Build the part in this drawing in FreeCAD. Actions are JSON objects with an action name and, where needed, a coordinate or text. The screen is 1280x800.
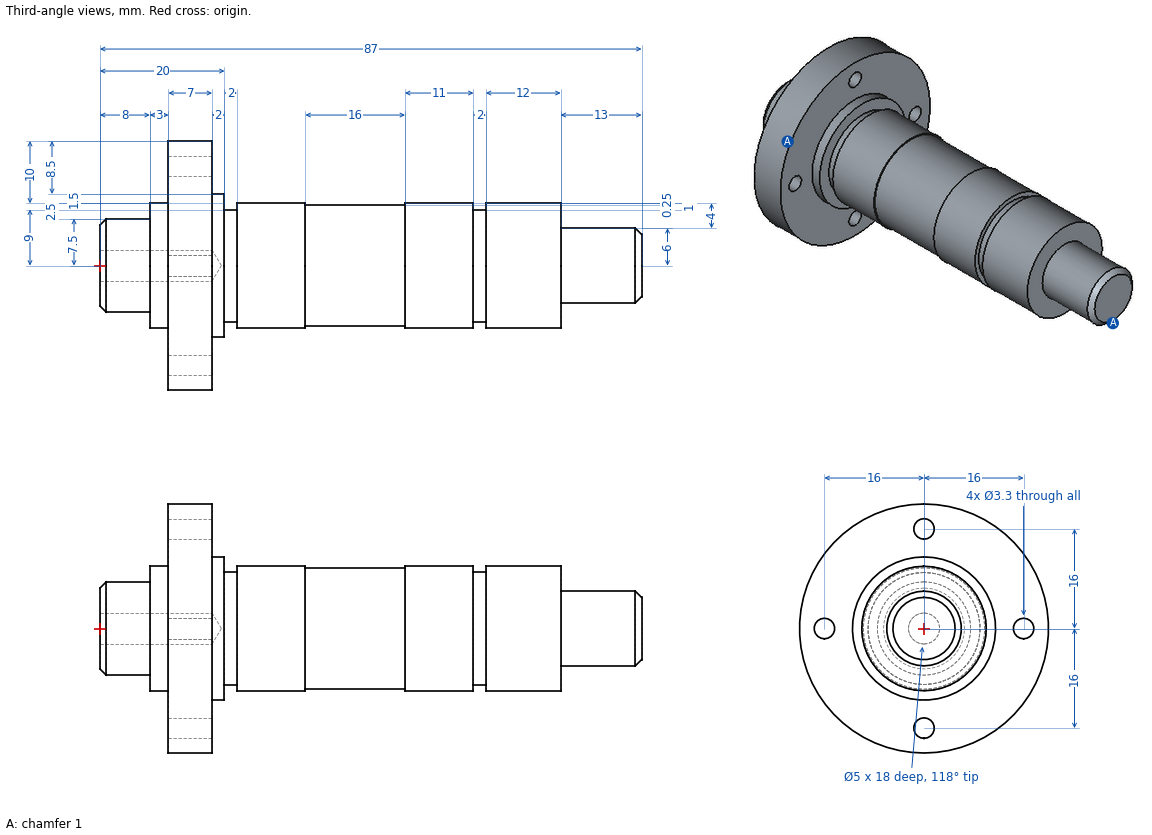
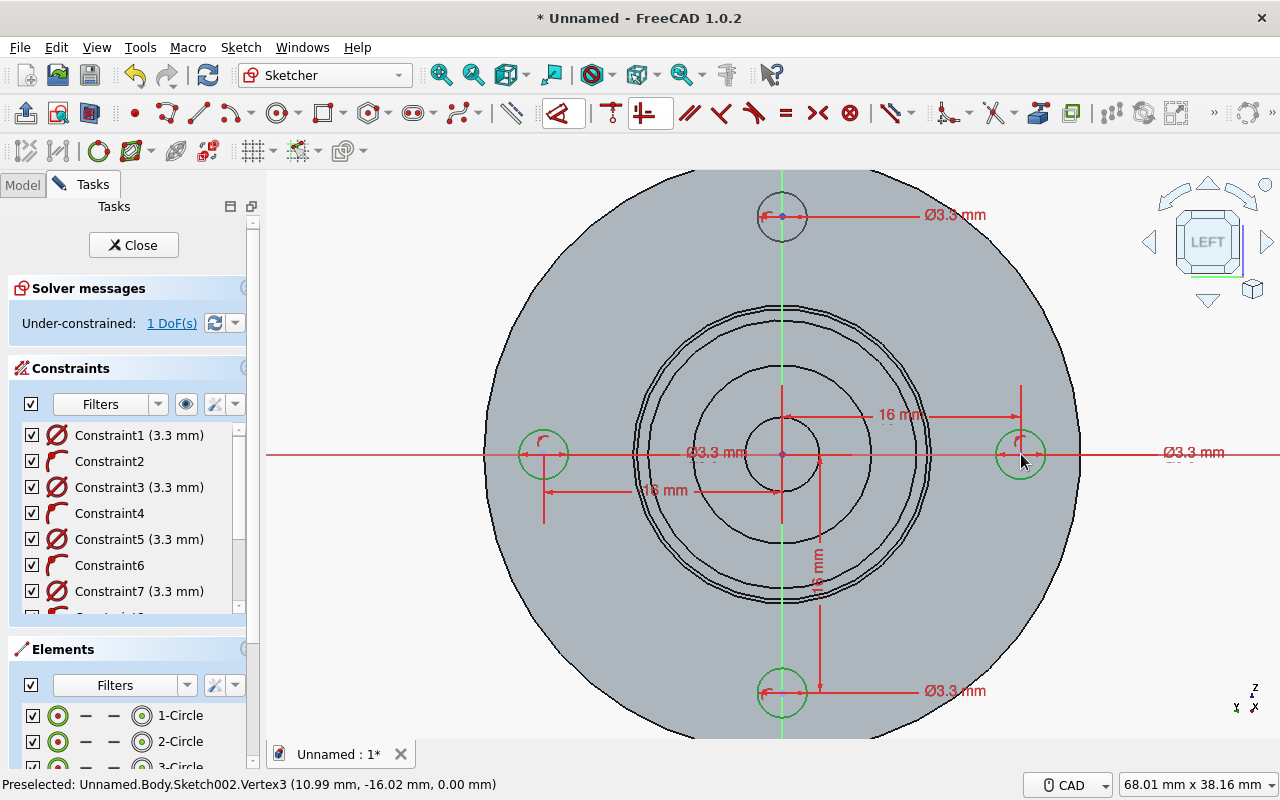
{"action": "left_click", "coordinate": [782, 217]}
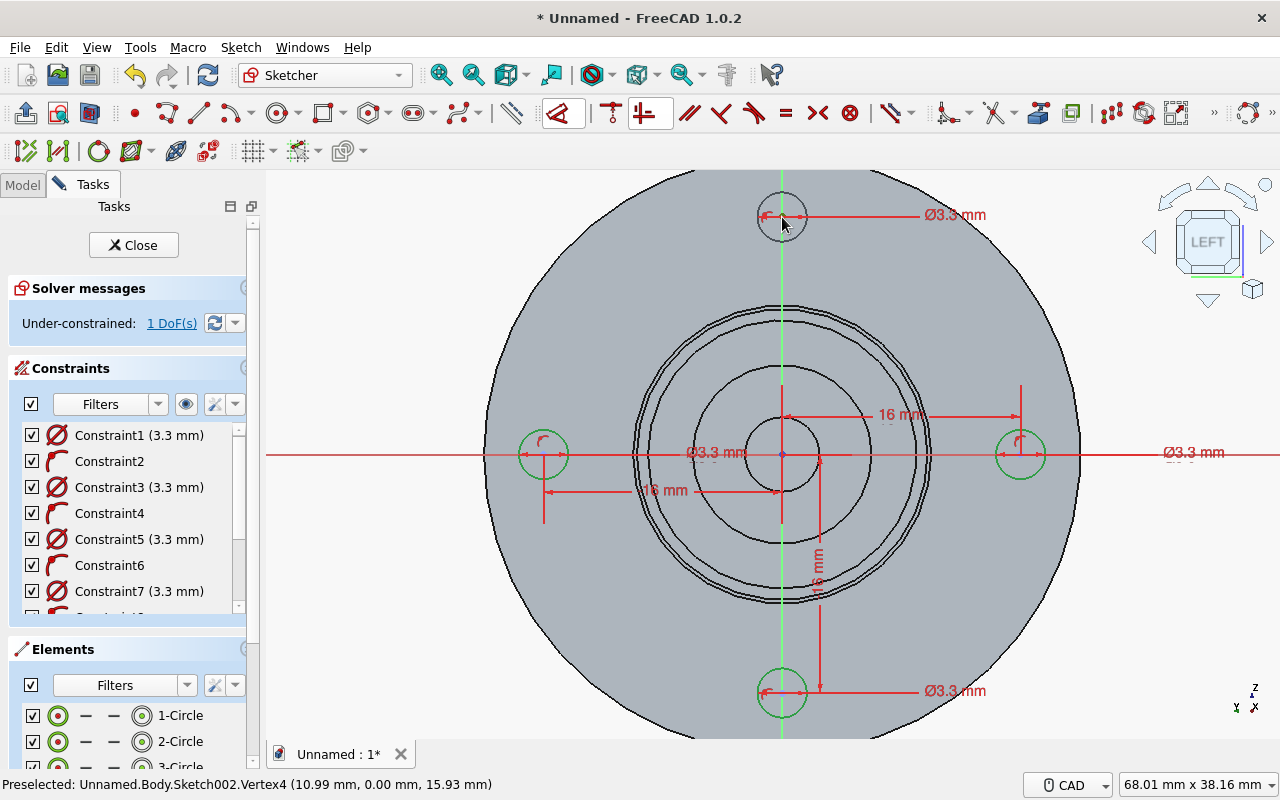
{"action": "key", "text": "i"}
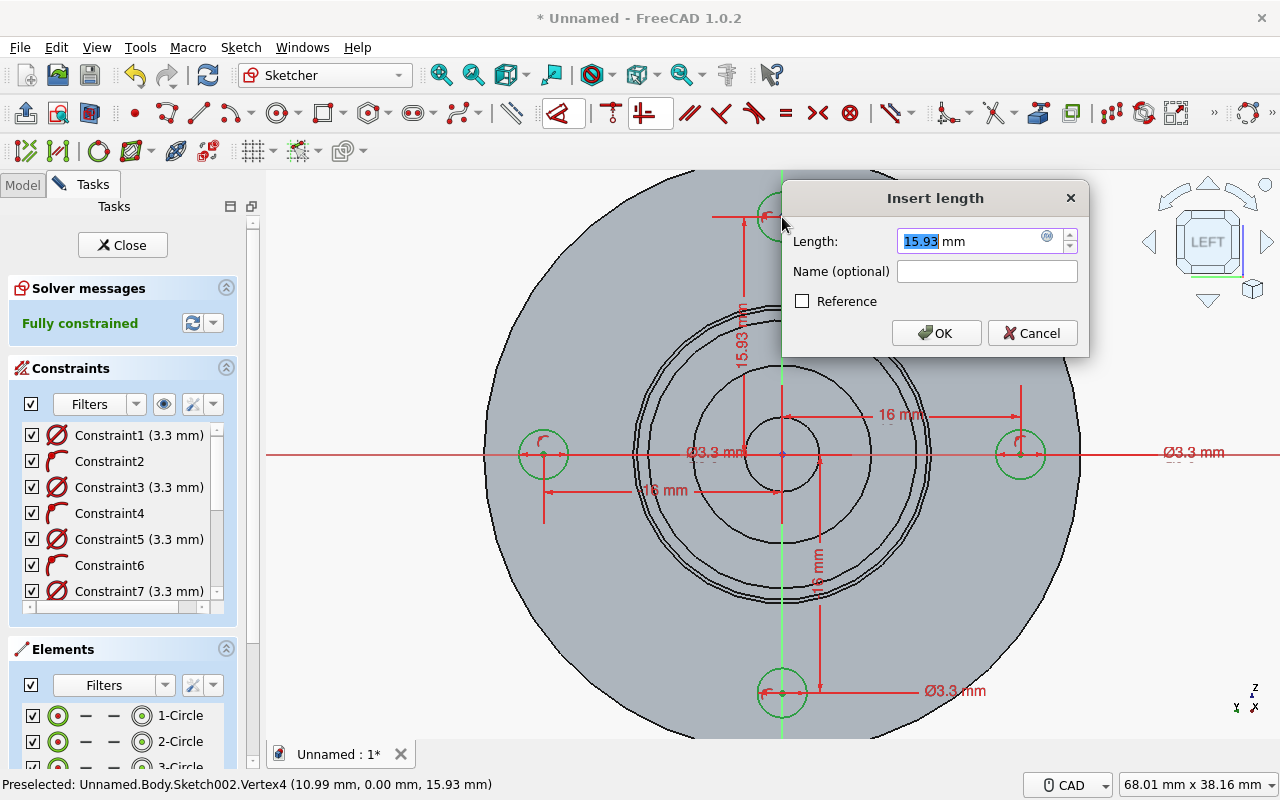
{"action": "type", "text": "16"}
{"action": "key", "text": "Return"}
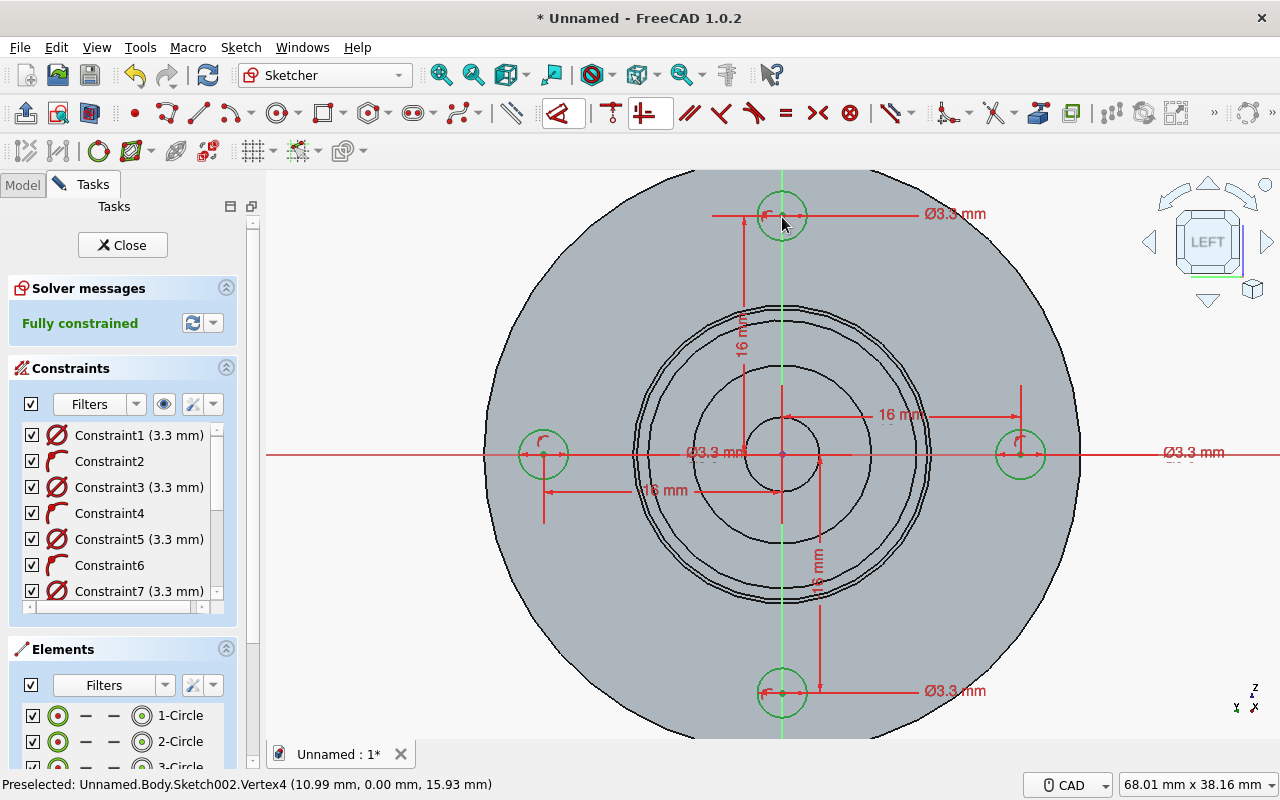
{"action": "left_click", "coordinate": [123, 245]}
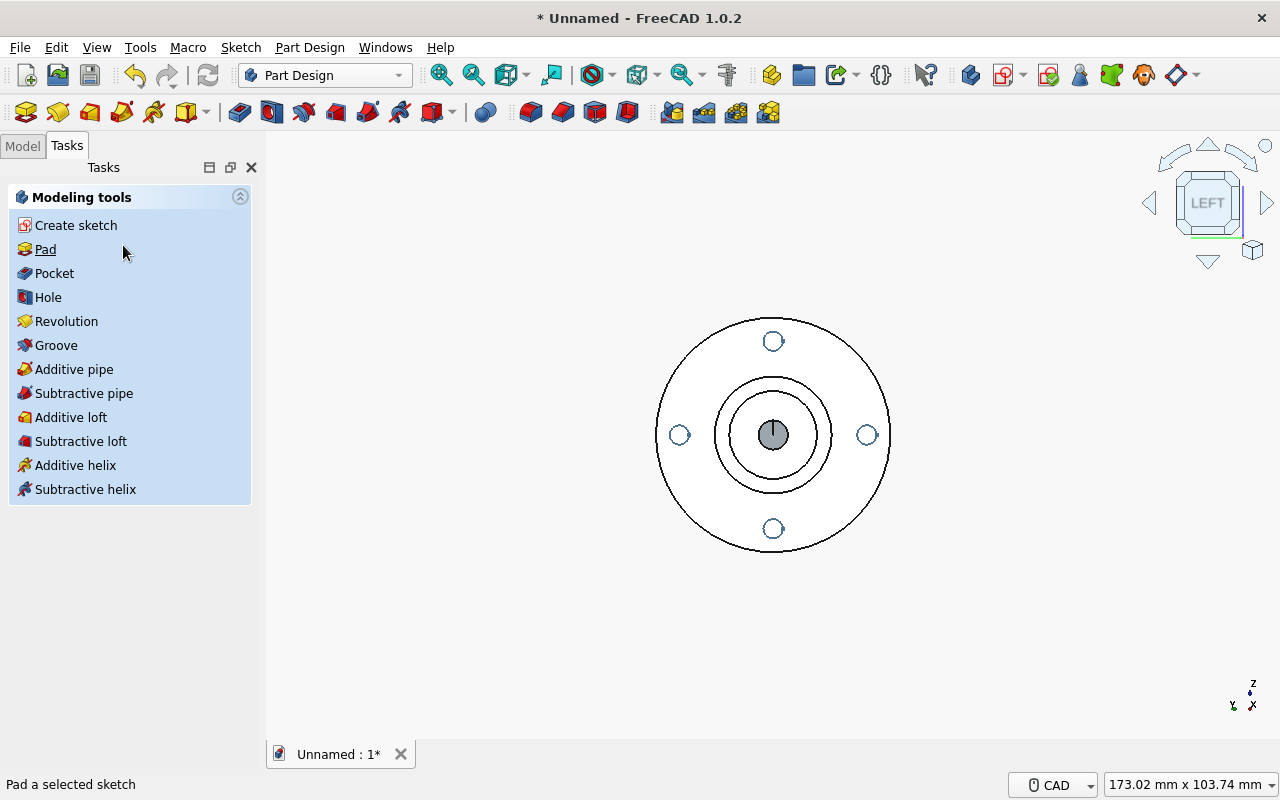
{"action": "left_click", "coordinate": [272, 112]}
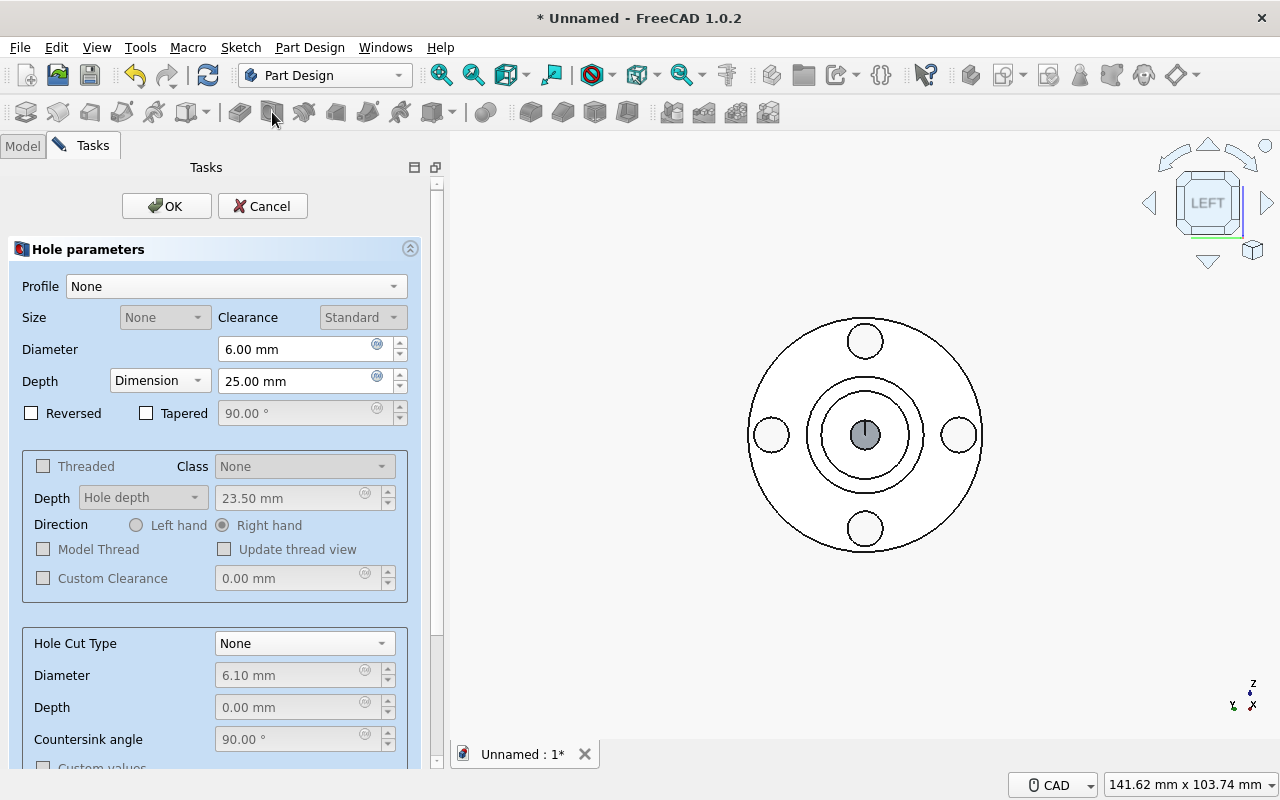
{"action": "triple_click", "coordinate": [305, 349]}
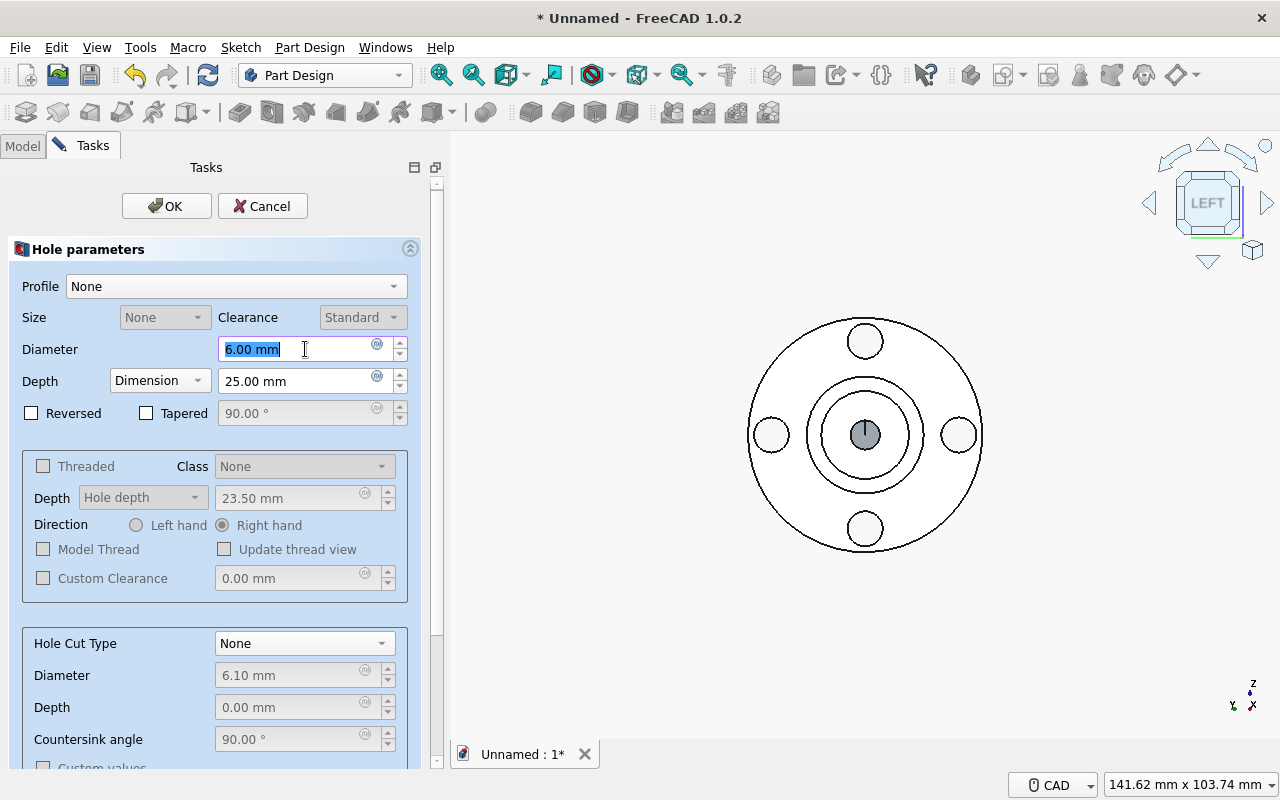
{"action": "type", "text": "3.3"}
{"action": "key", "text": "Tab"}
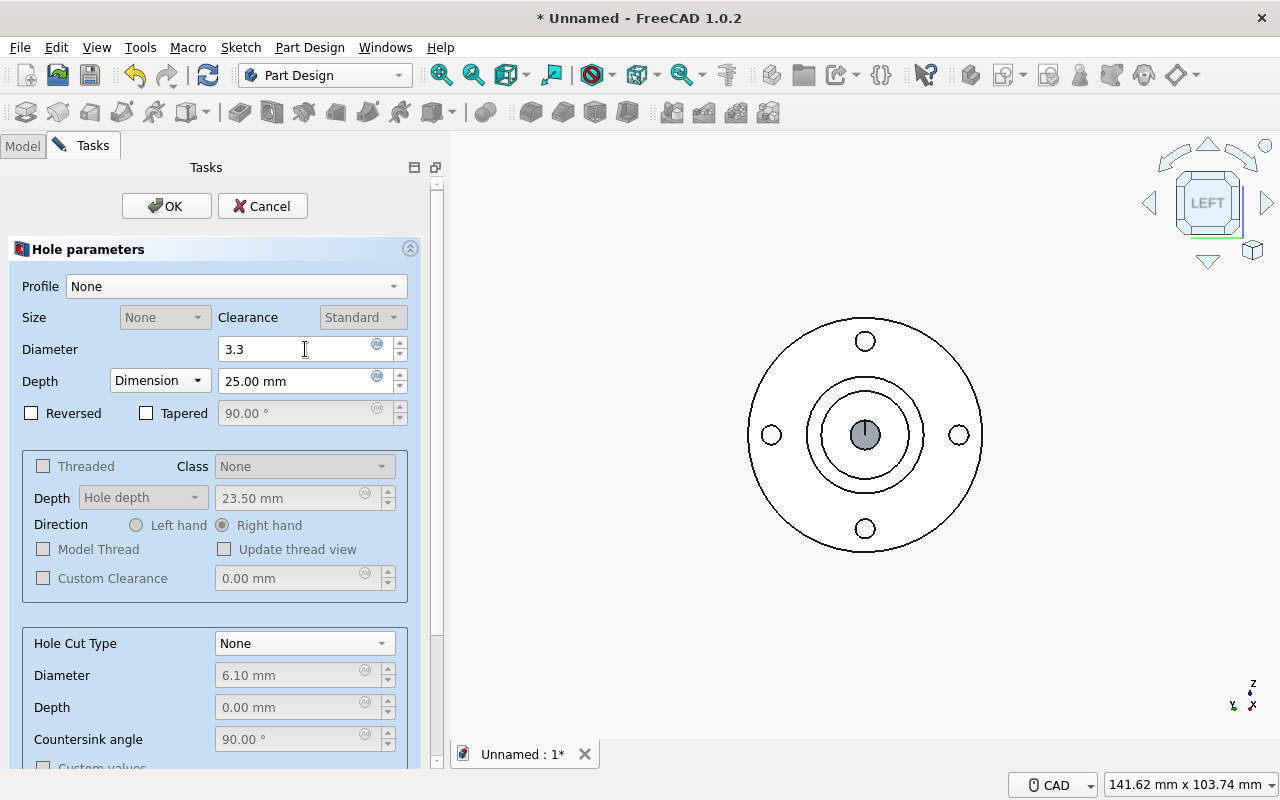
{"action": "left_click", "coordinate": [161, 380]}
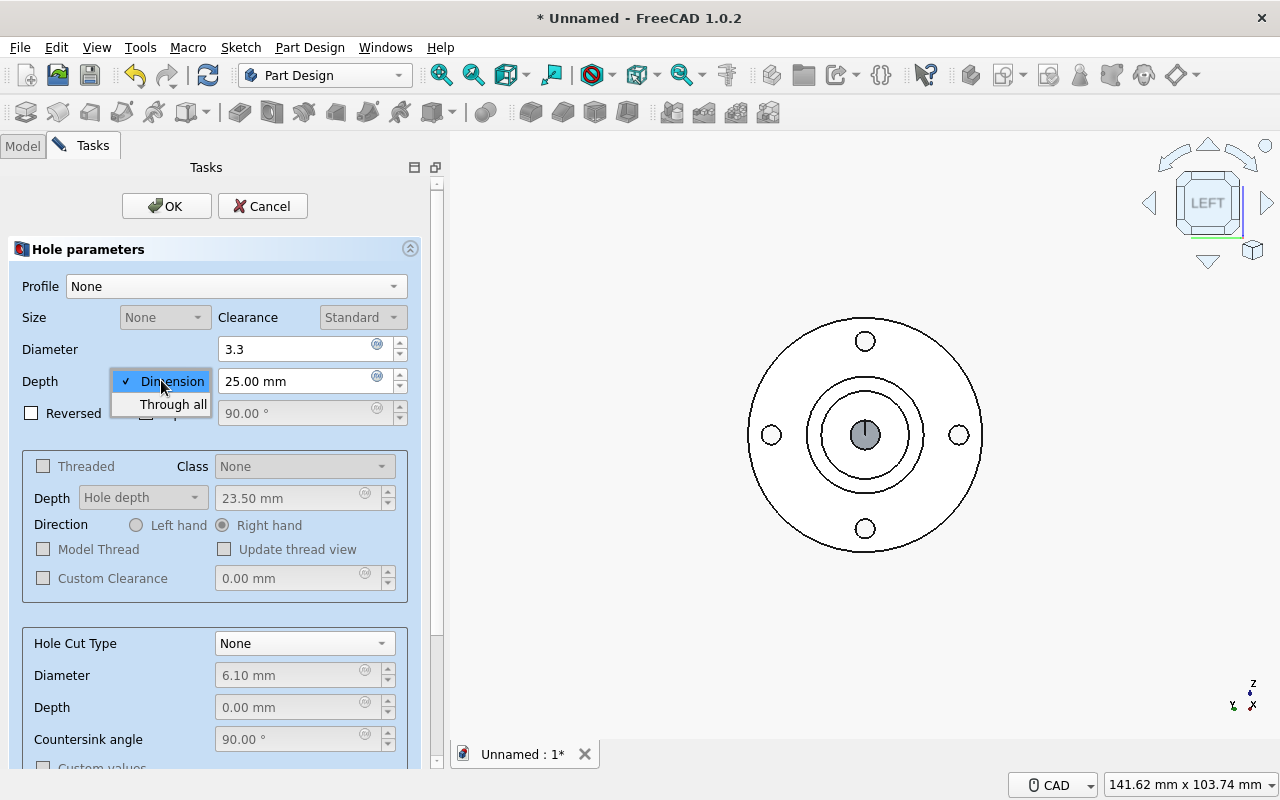
{"action": "left_click", "coordinate": [160, 404]}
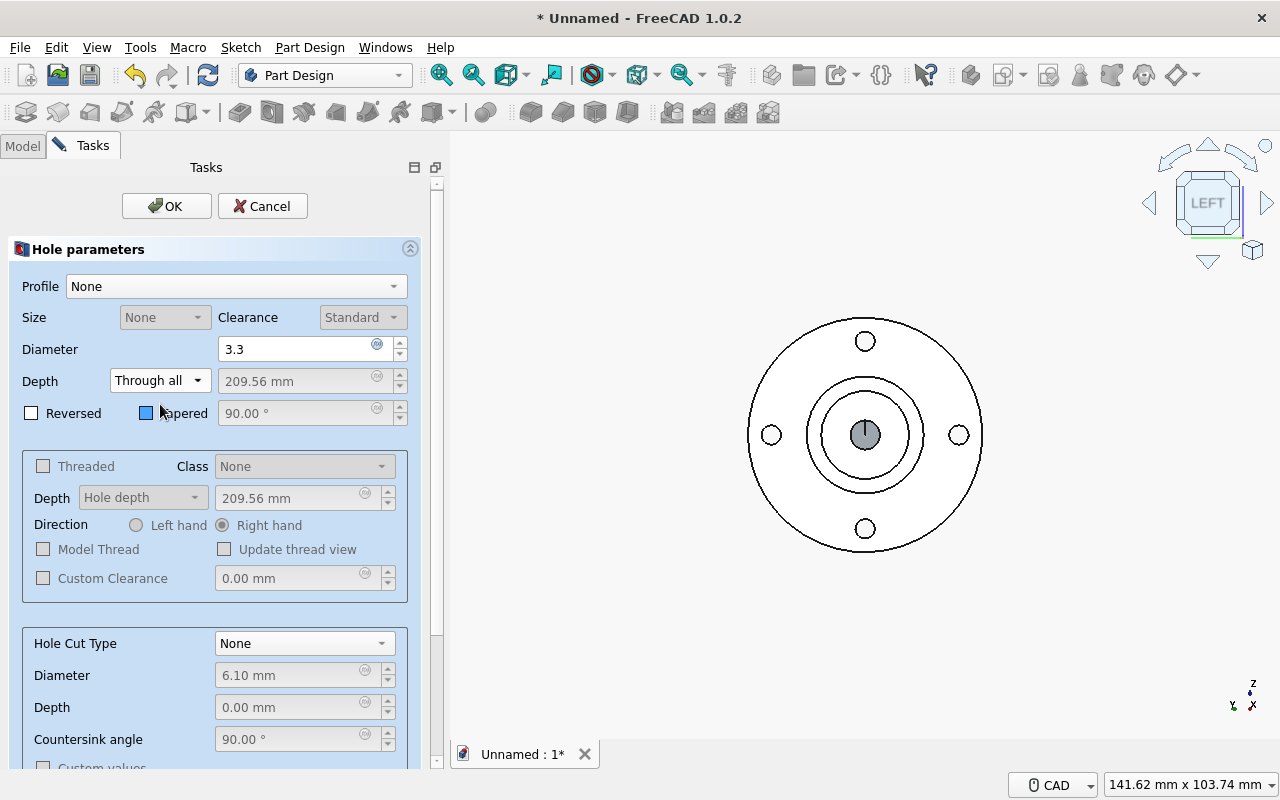
{"action": "left_click", "coordinate": [167, 206]}